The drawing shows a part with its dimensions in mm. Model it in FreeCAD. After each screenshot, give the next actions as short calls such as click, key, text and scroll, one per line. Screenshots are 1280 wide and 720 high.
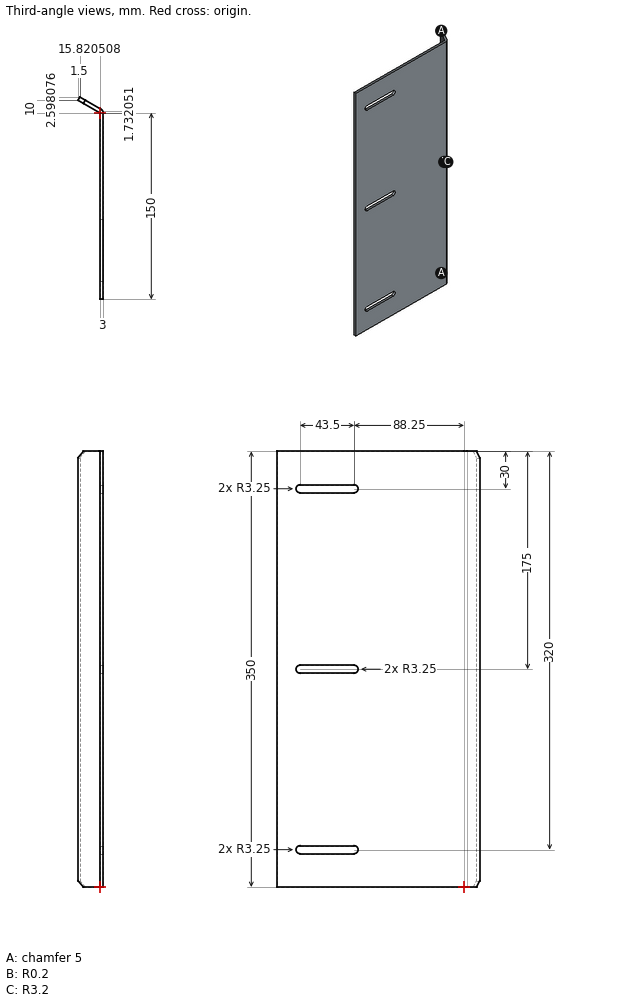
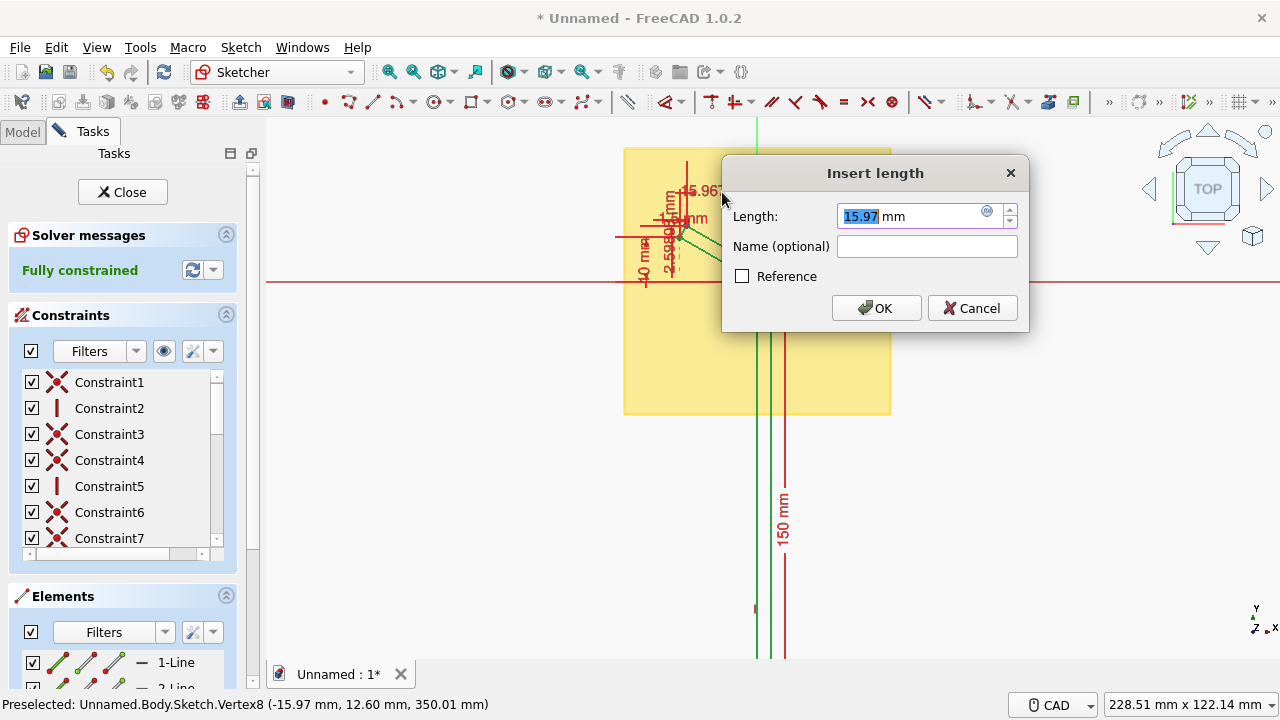
text(15.820508)
key(Return)
key(Escape)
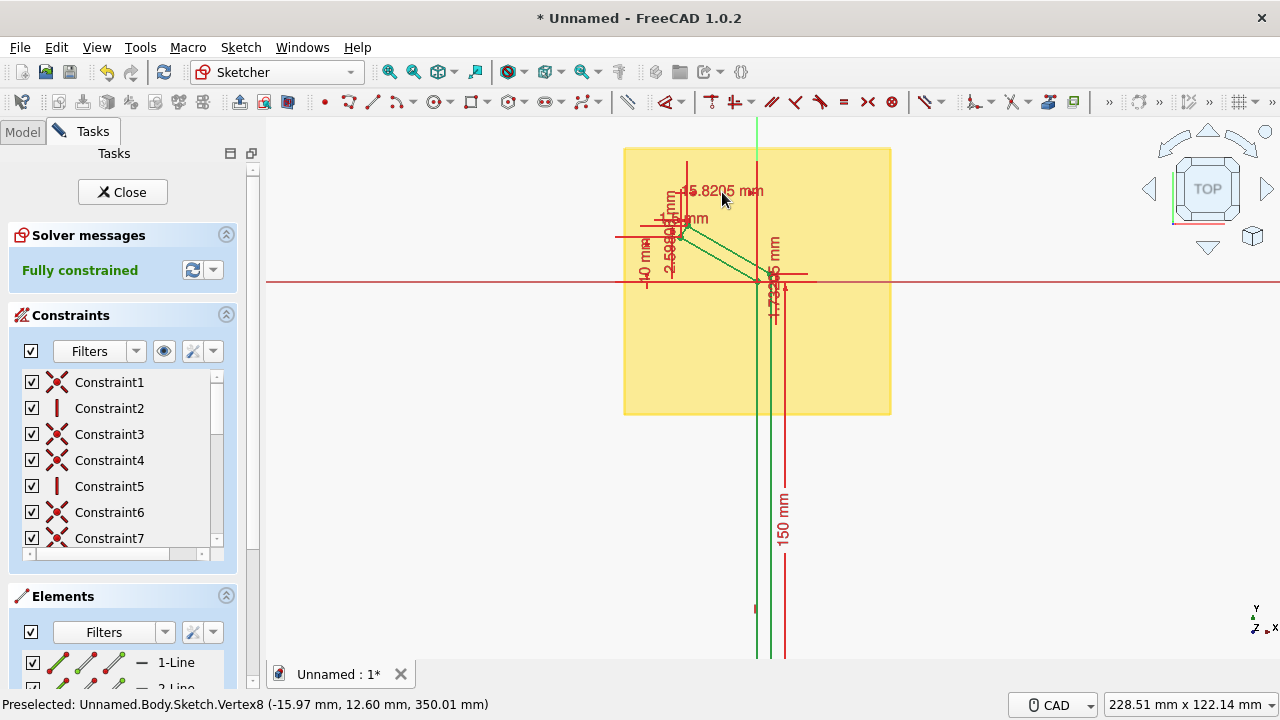
click(123, 192)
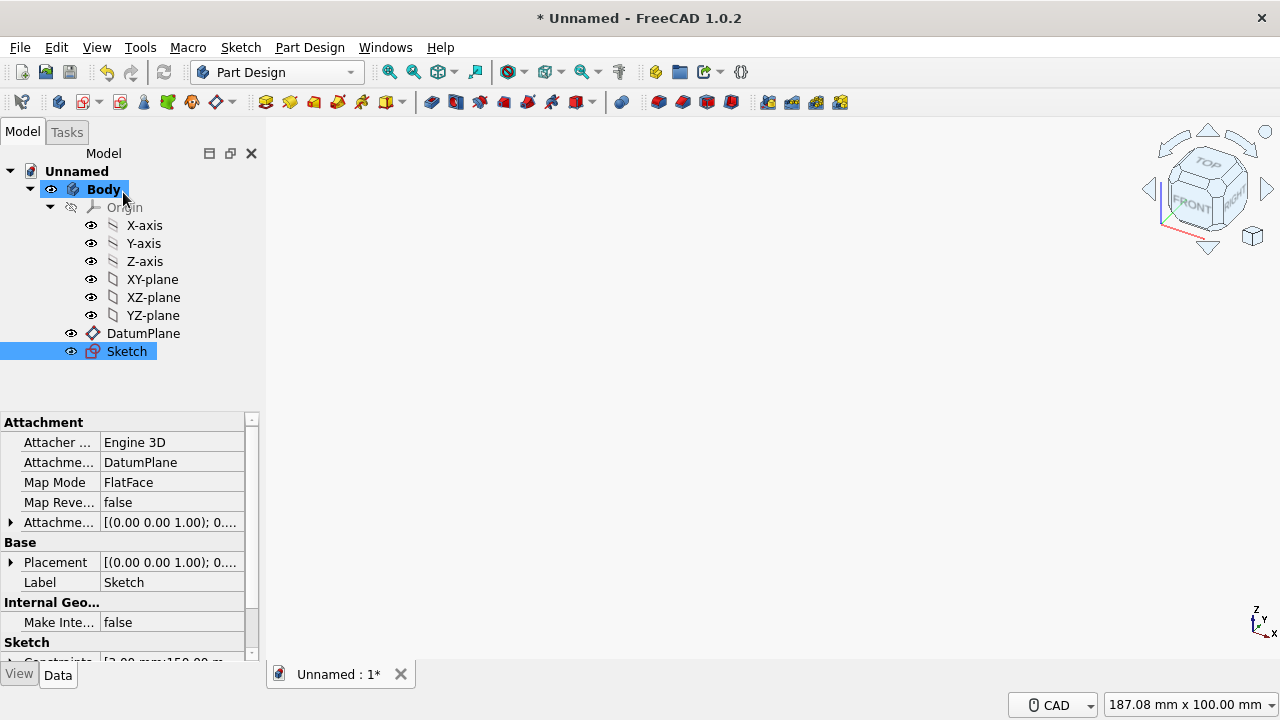
click(266, 102)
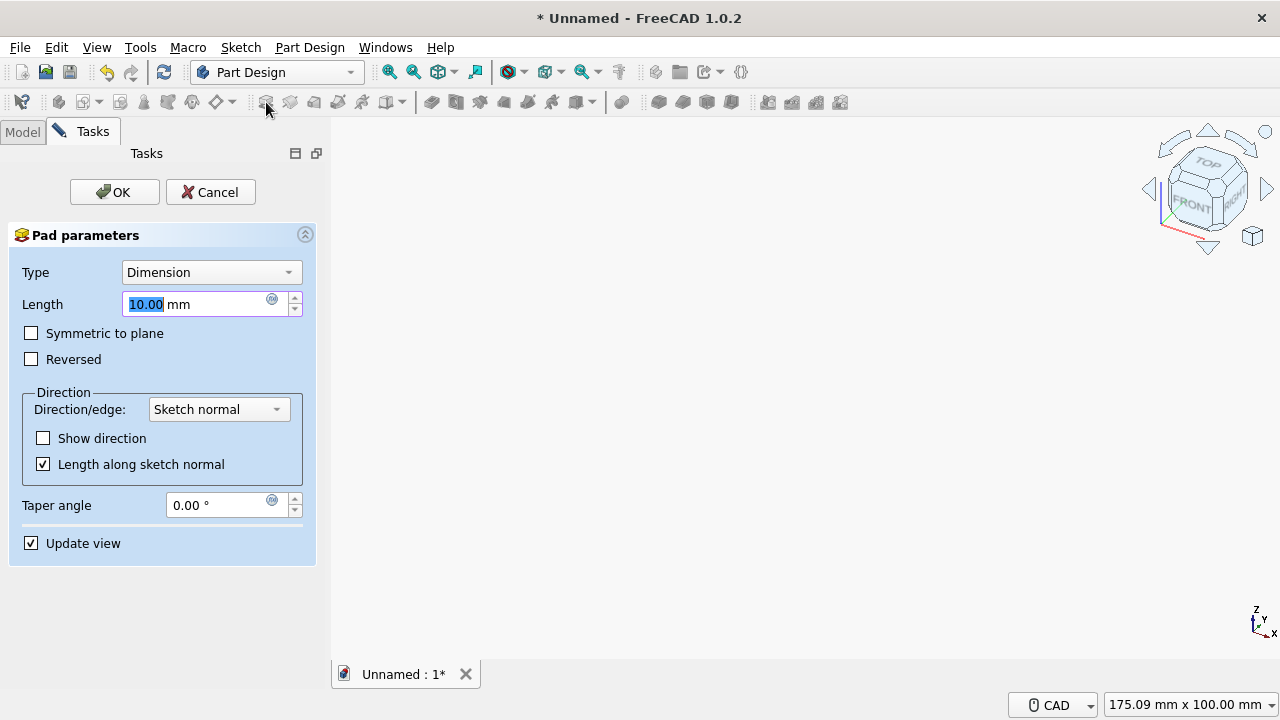
text(350)
key(Tab)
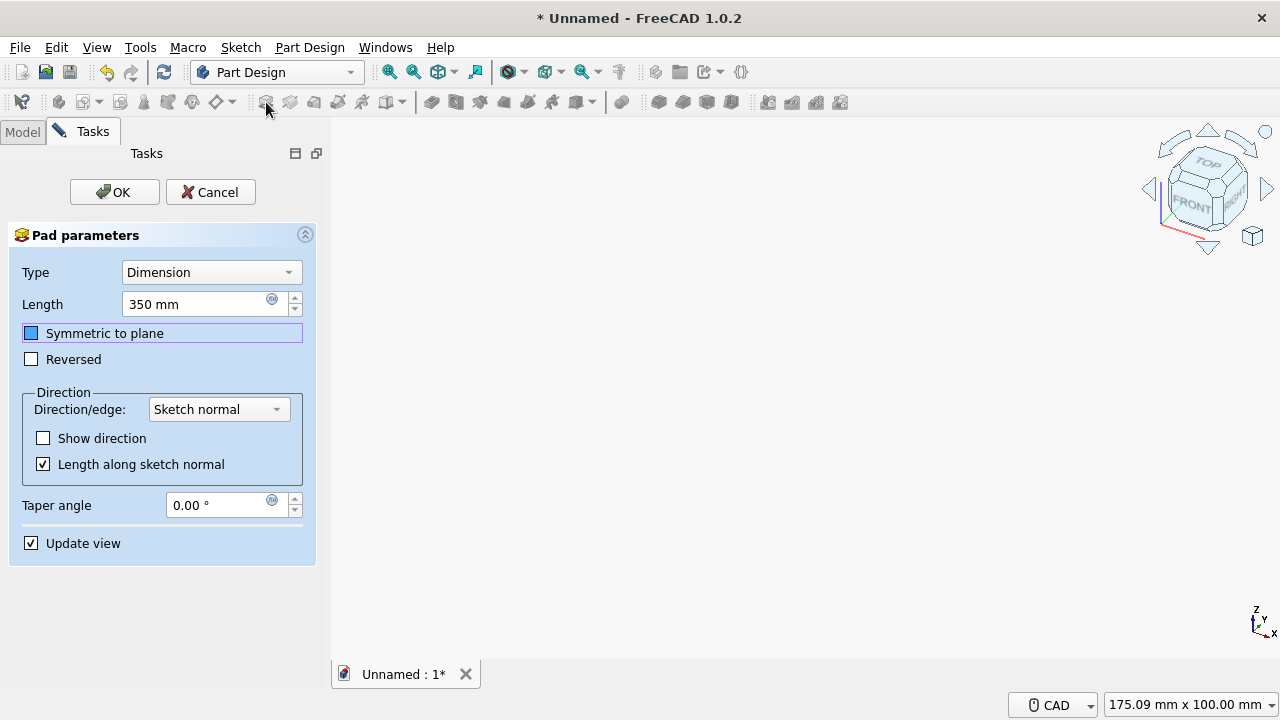
click(30, 359)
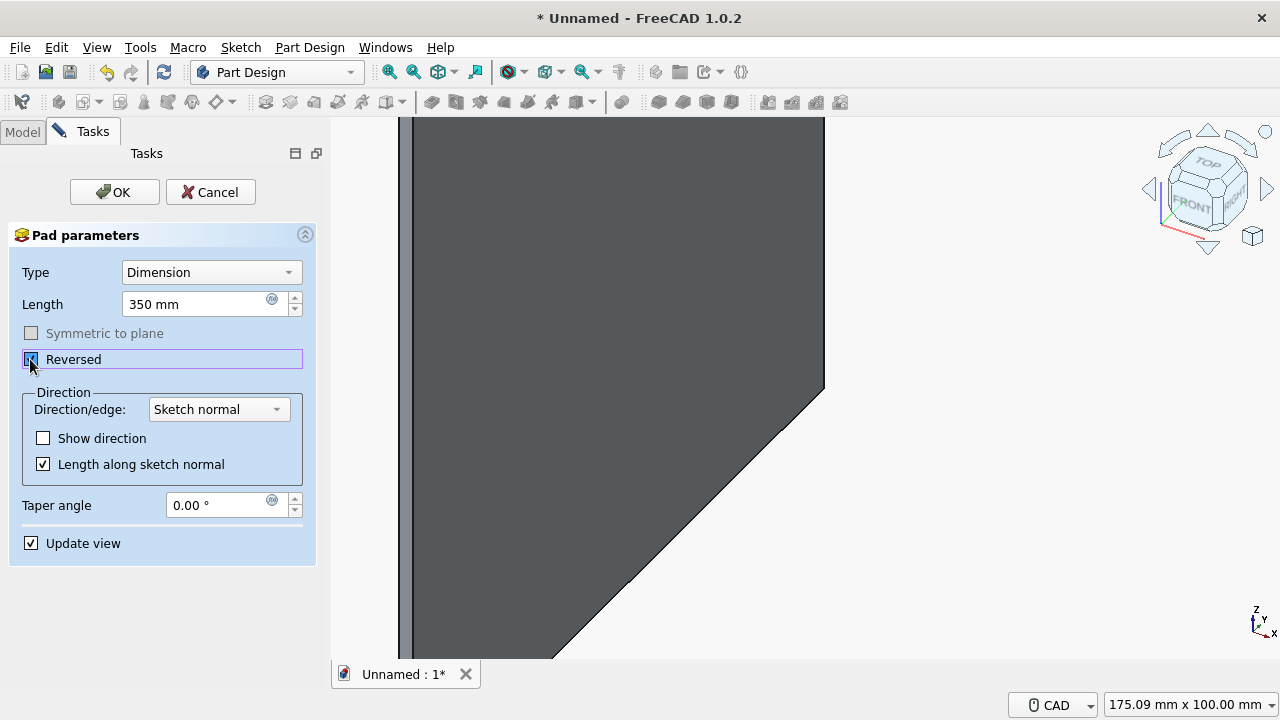
click(115, 192)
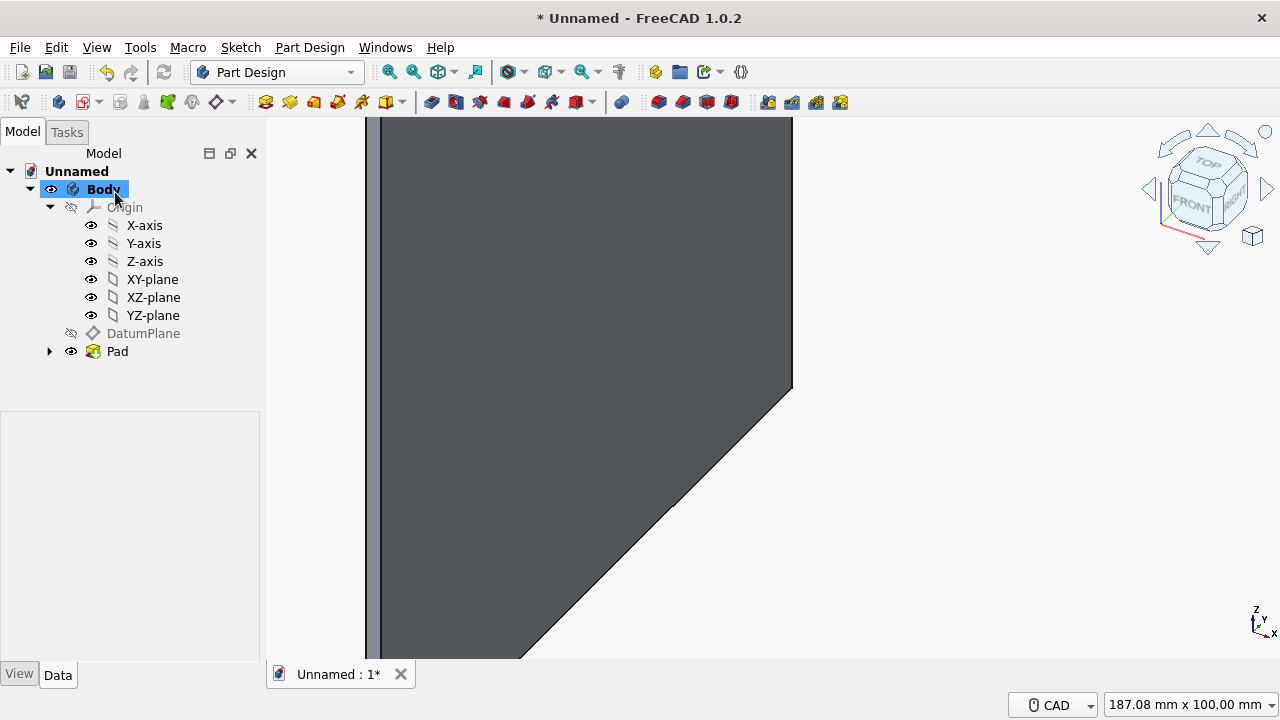
click(390, 72)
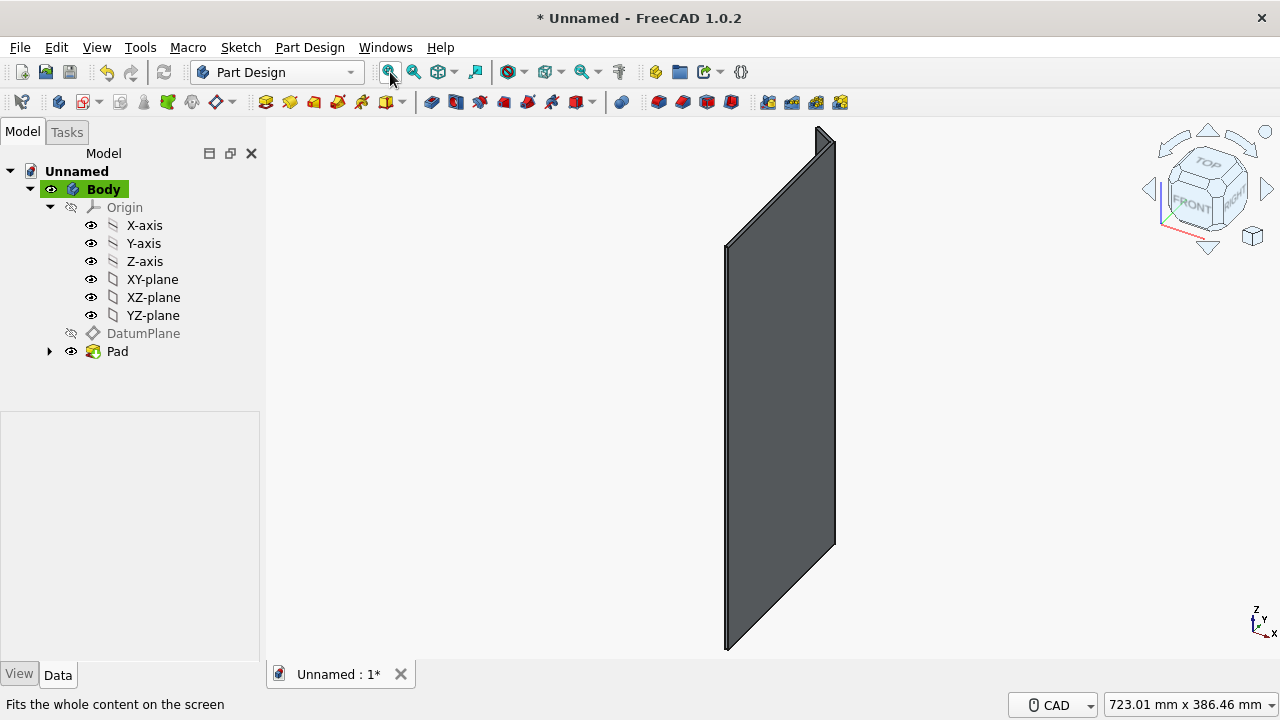
key(6)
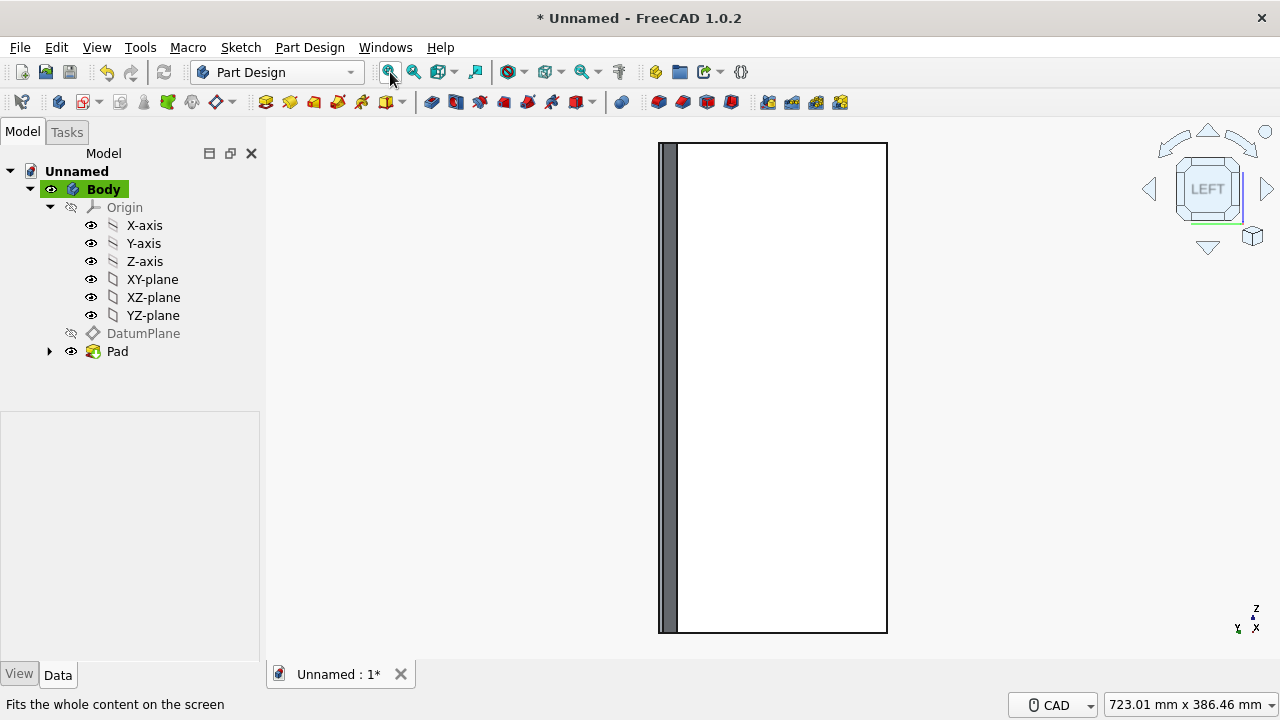
click(782, 247)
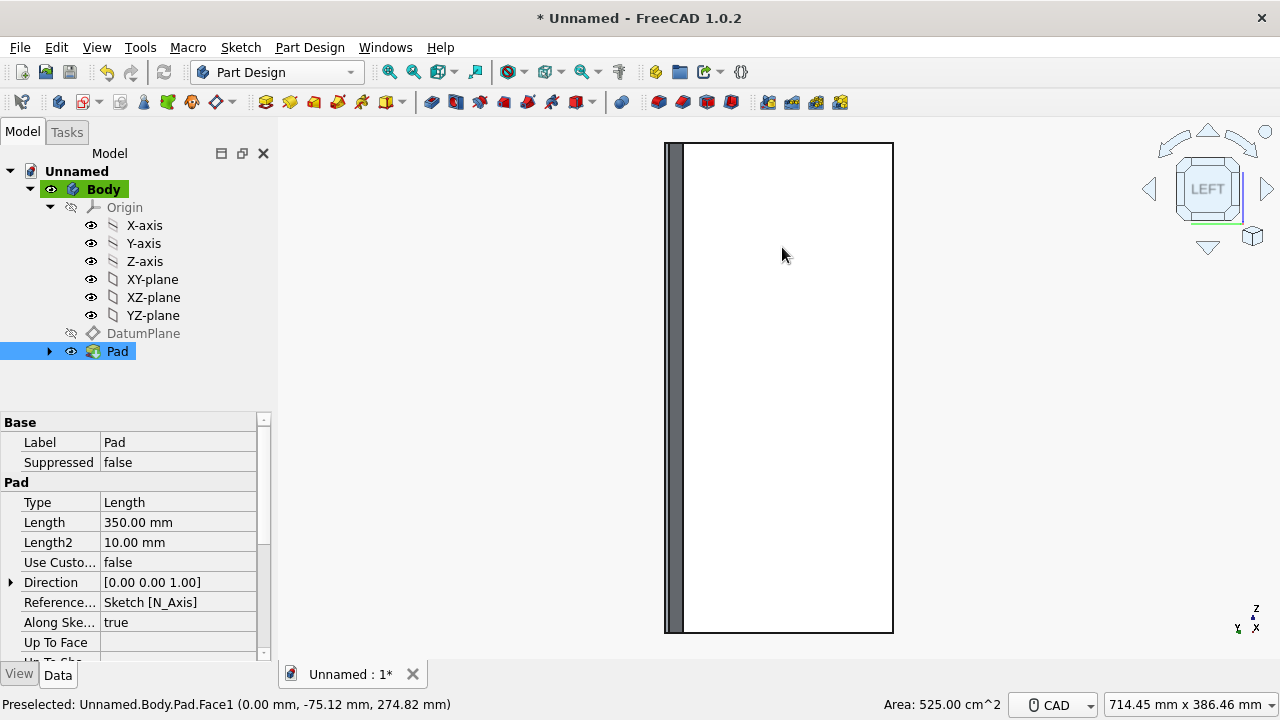
click(84, 102)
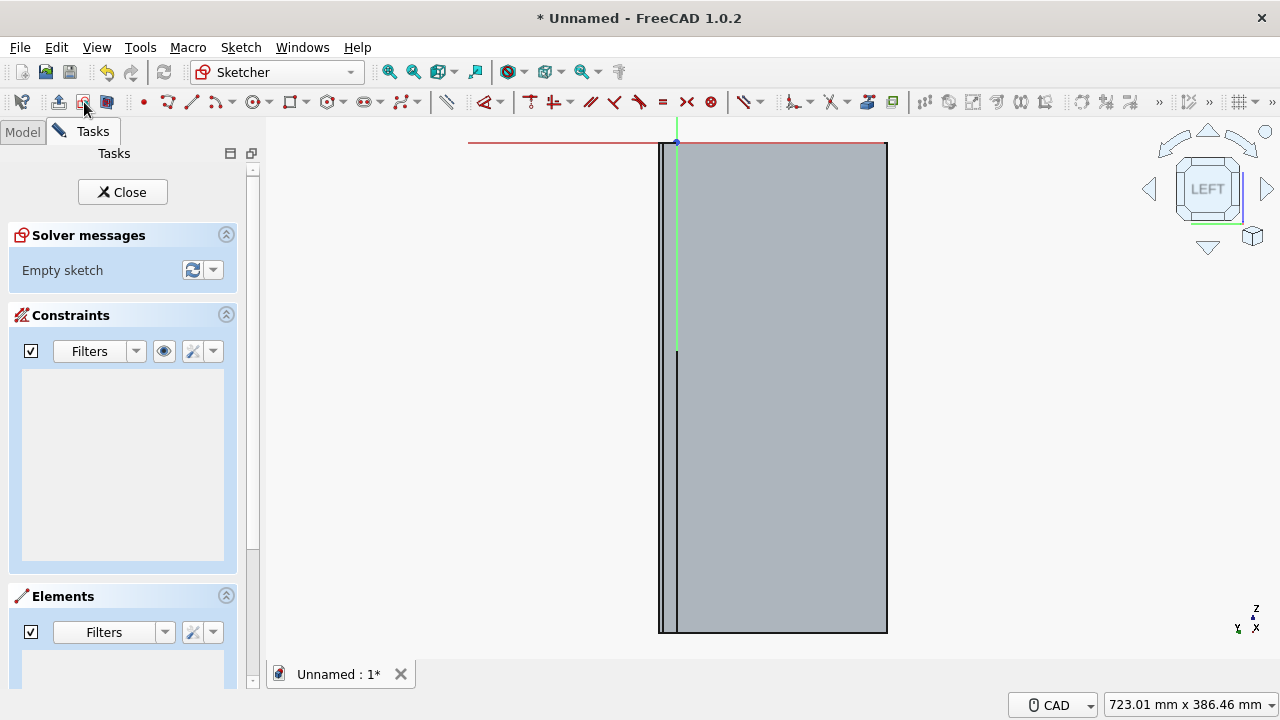
key(q)
key(s)